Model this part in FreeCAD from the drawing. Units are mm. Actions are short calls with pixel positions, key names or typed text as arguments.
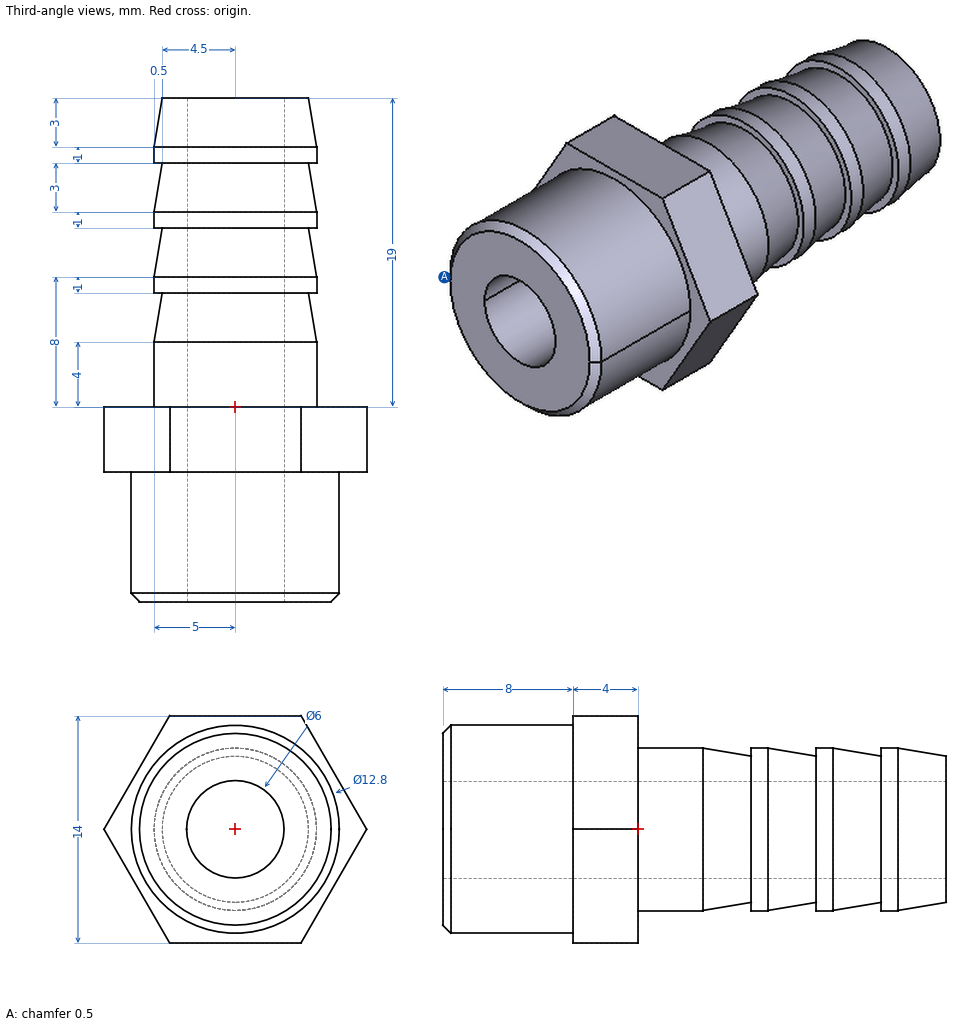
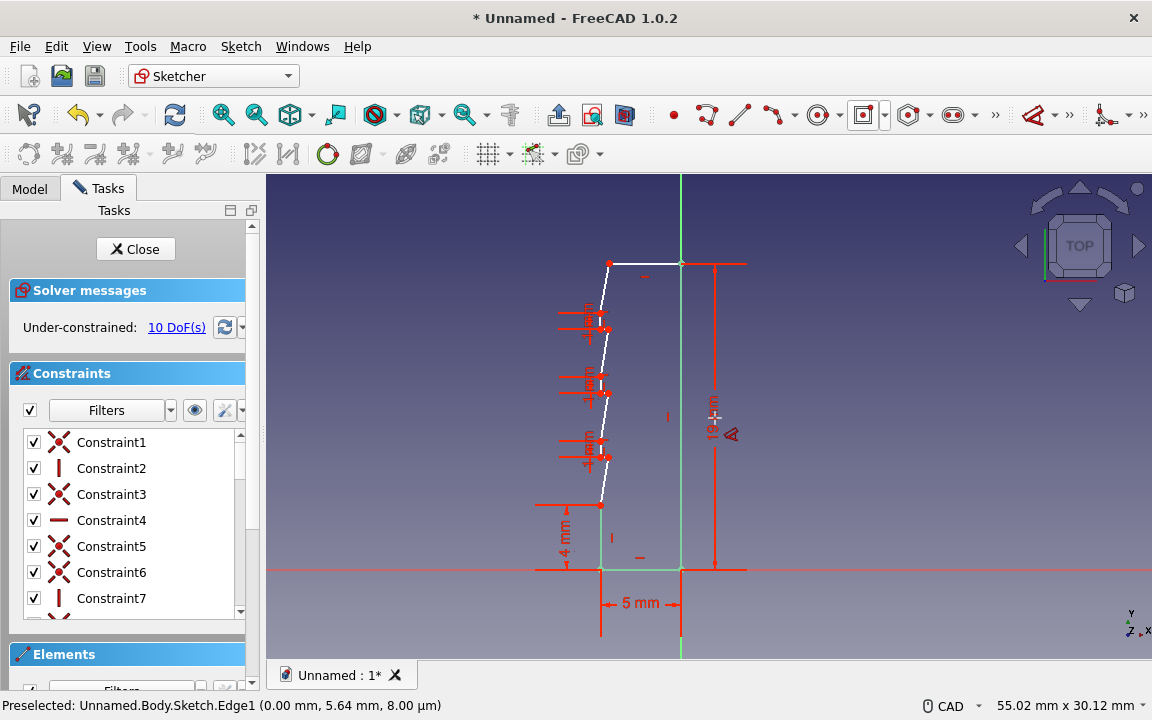
click(600, 313)
click(641, 279)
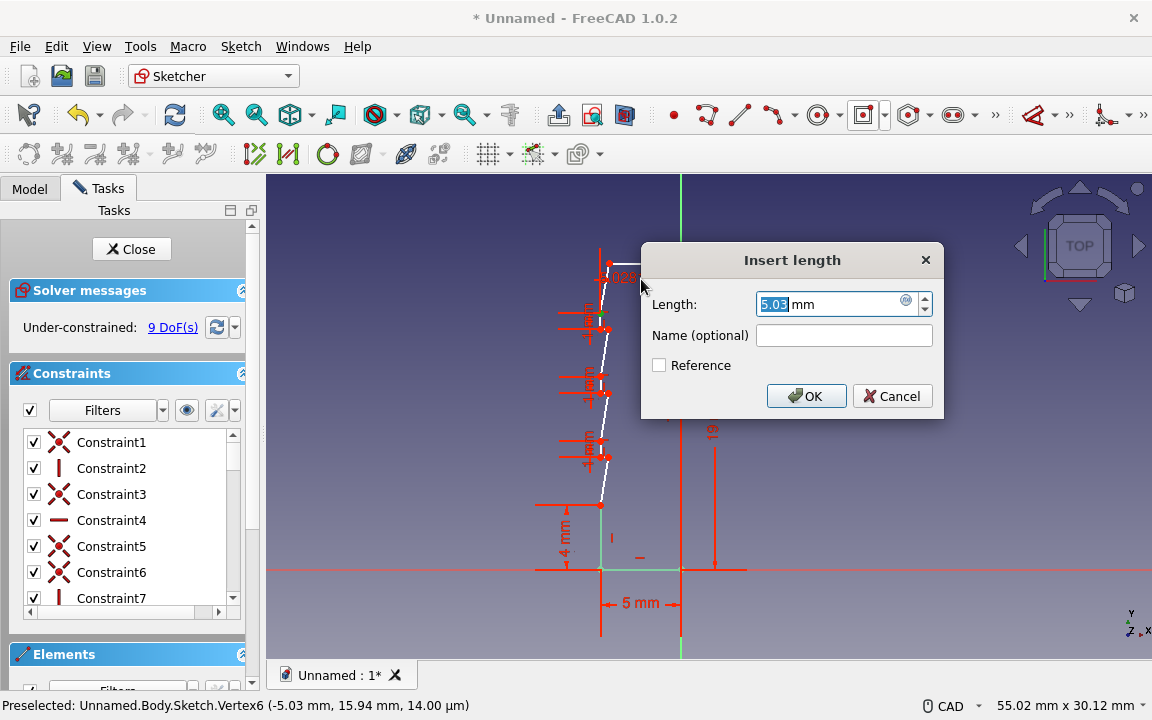
text(5)
key(Return)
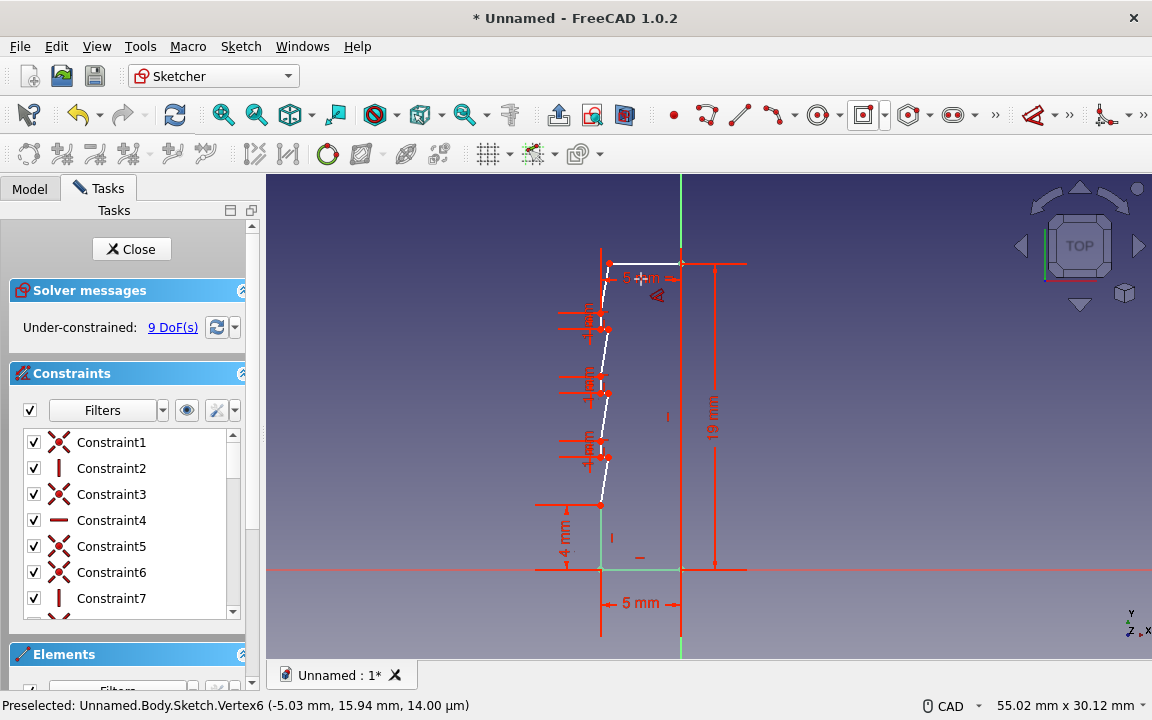
click(601, 377)
click(641, 343)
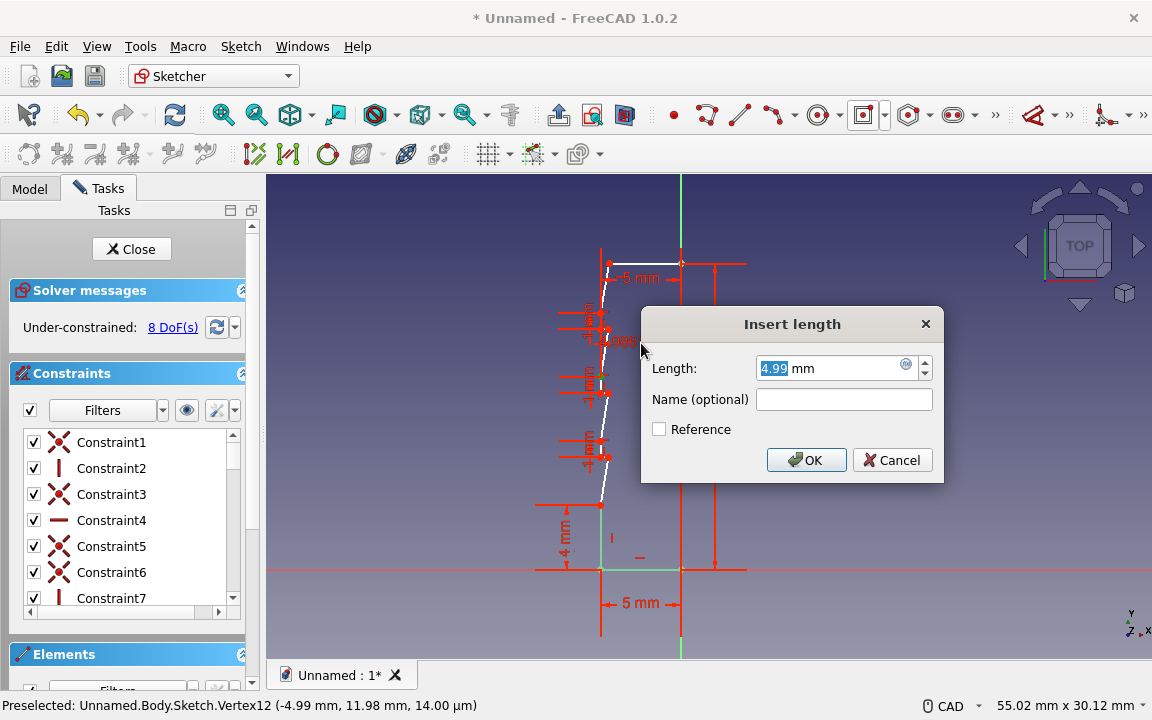
text(5)
key(Return)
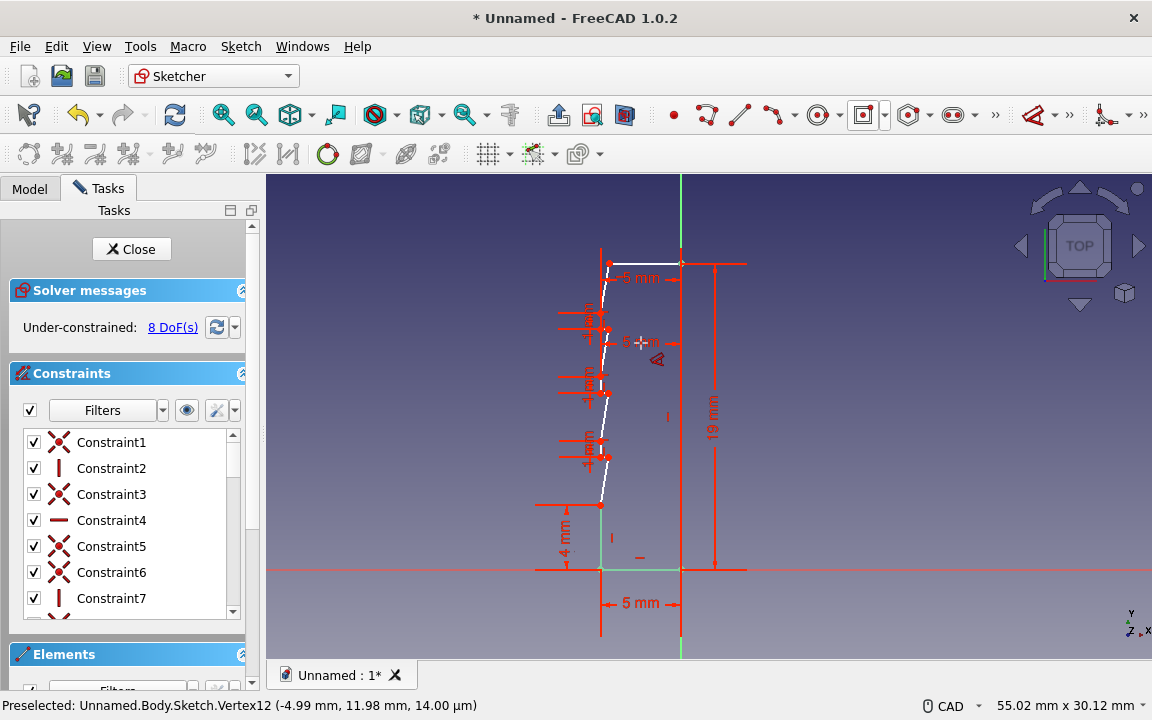
click(601, 441)
click(641, 407)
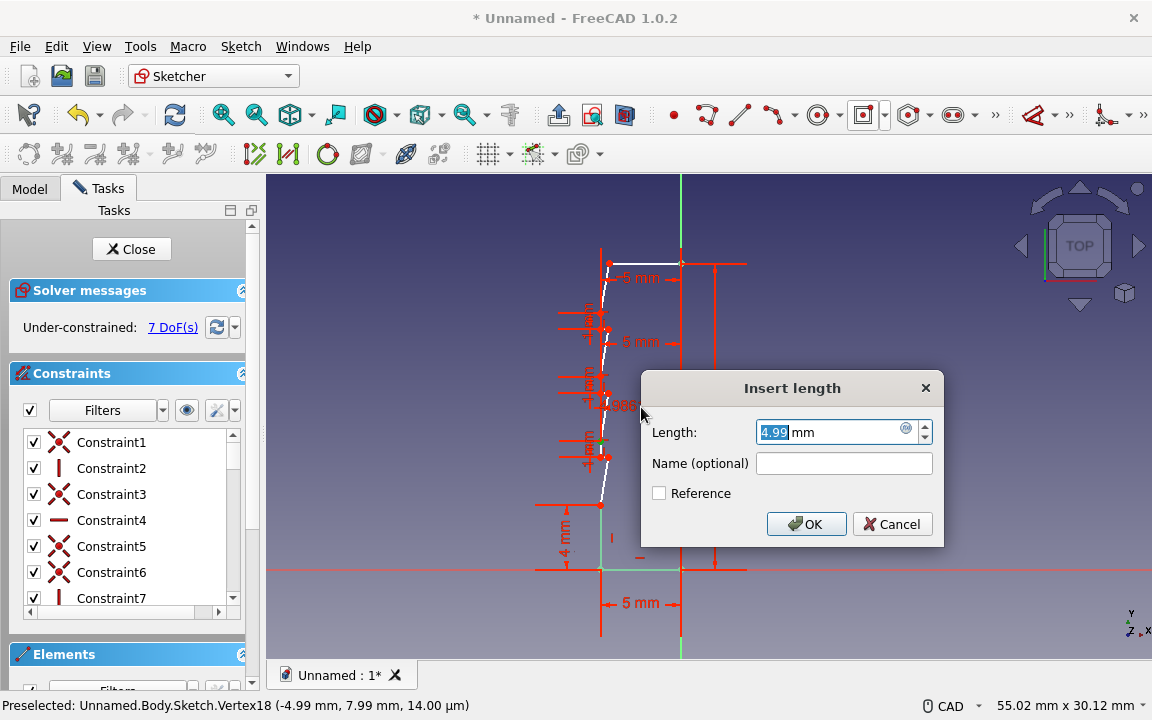
text(5)
key(Return)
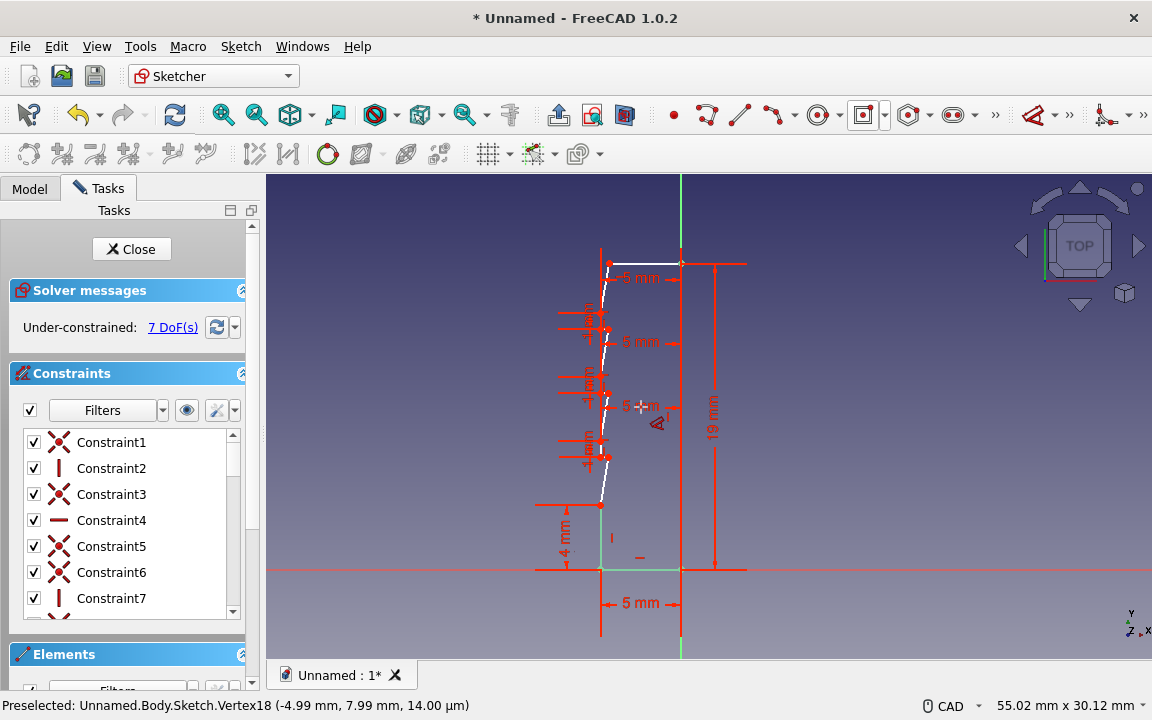
click(601, 441)
click(715, 506)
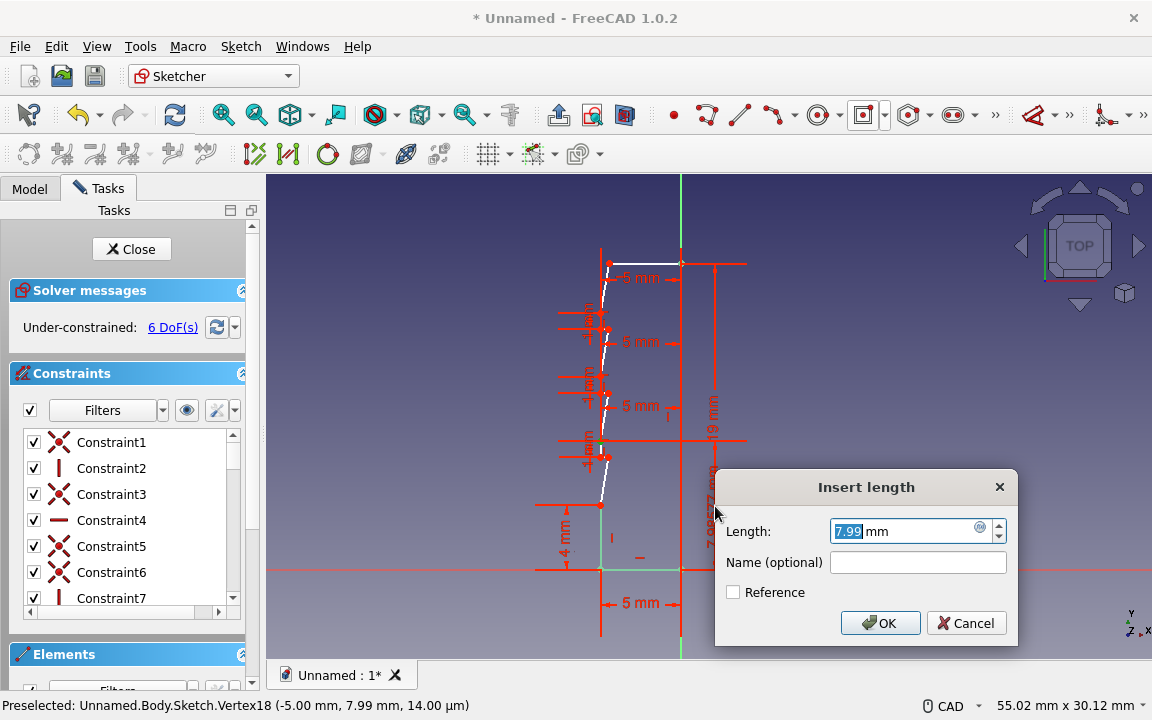
text(8)
key(Return)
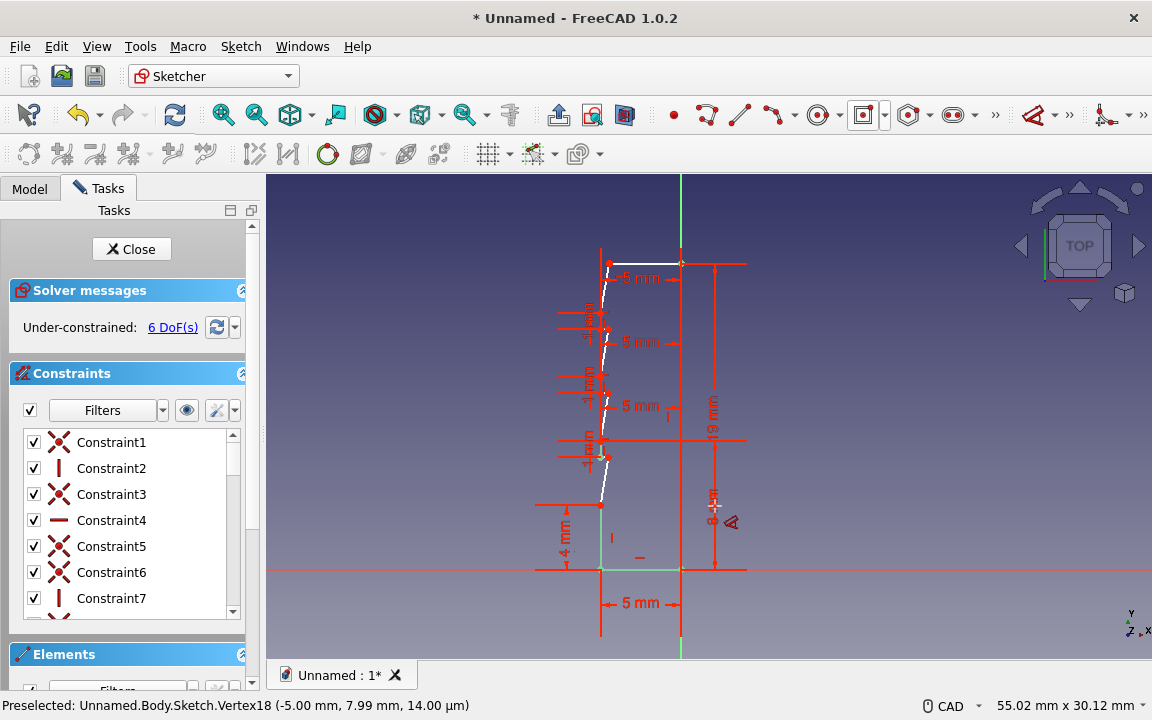
click(607, 279)
click(567, 288)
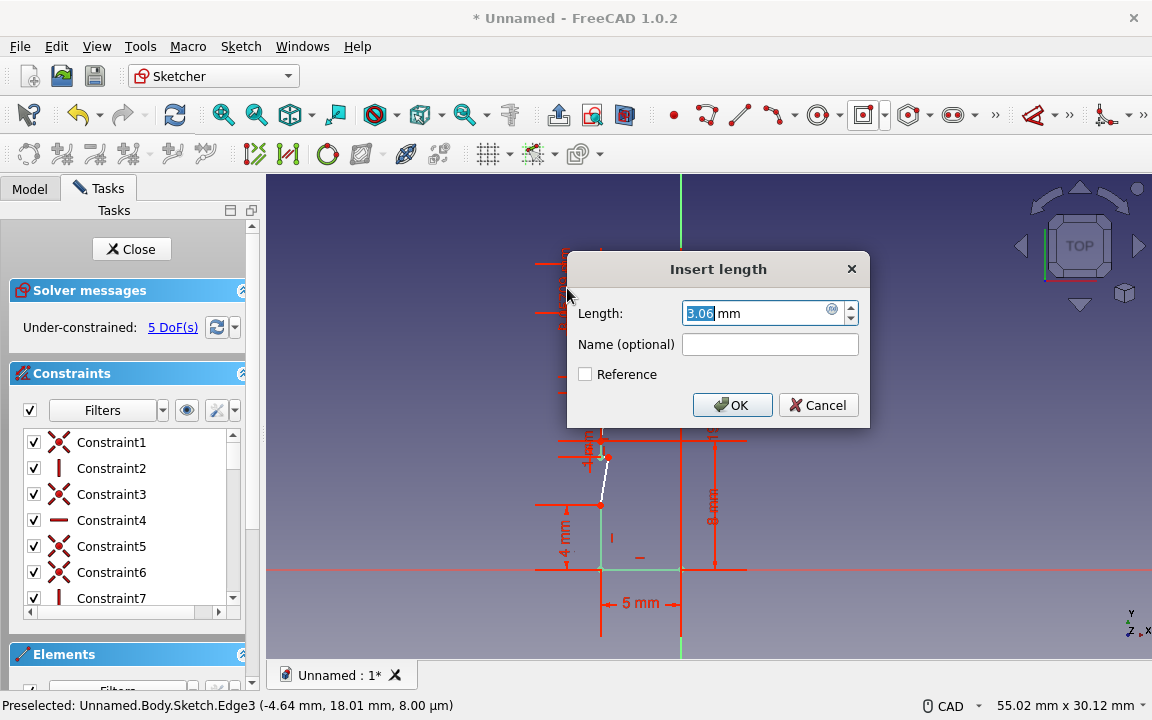
text(3)
key(Return)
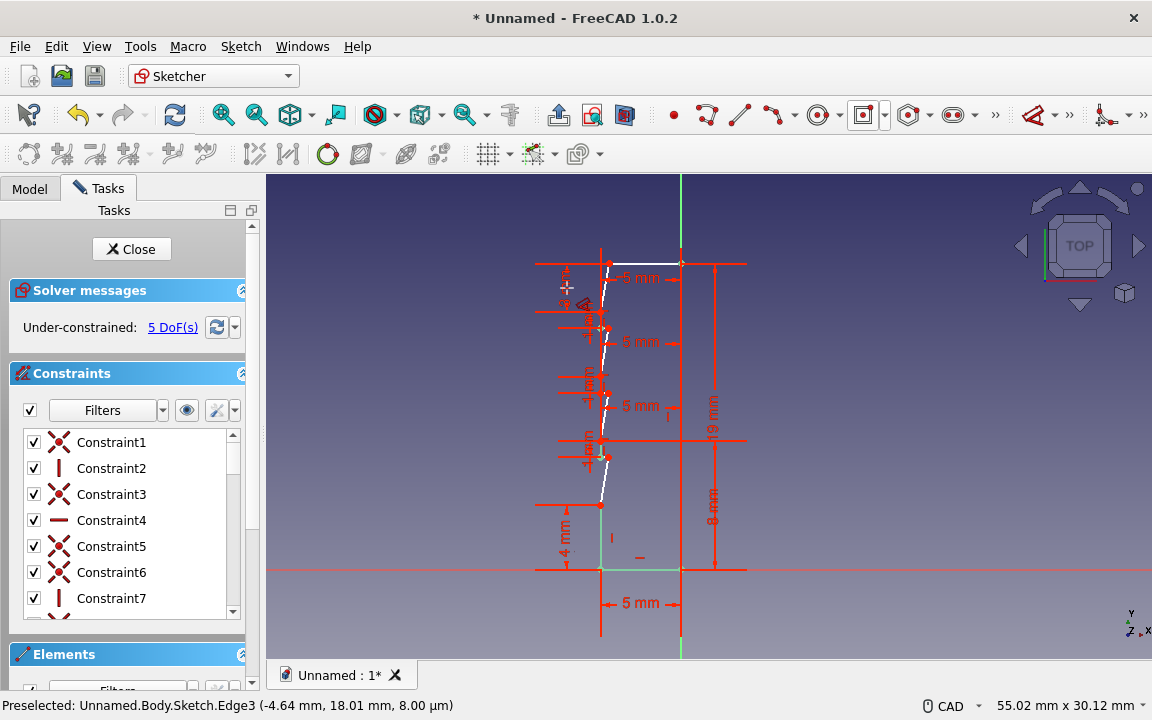
click(606, 343)
click(567, 353)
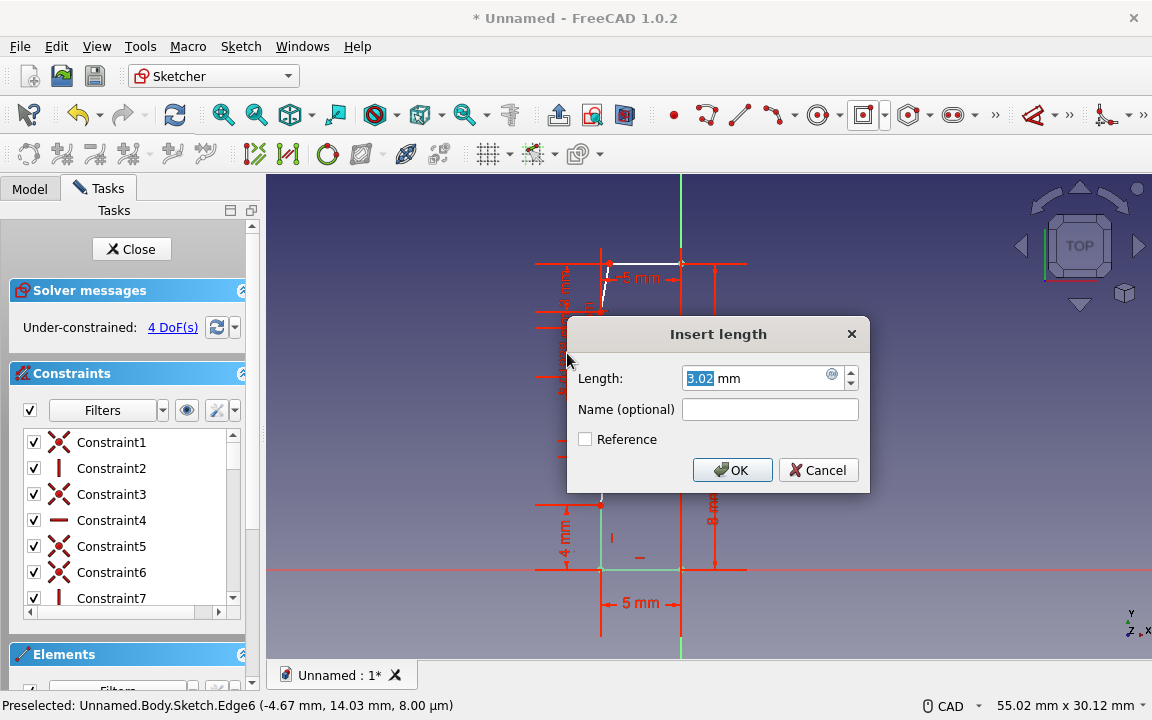
text(3)
key(Return)